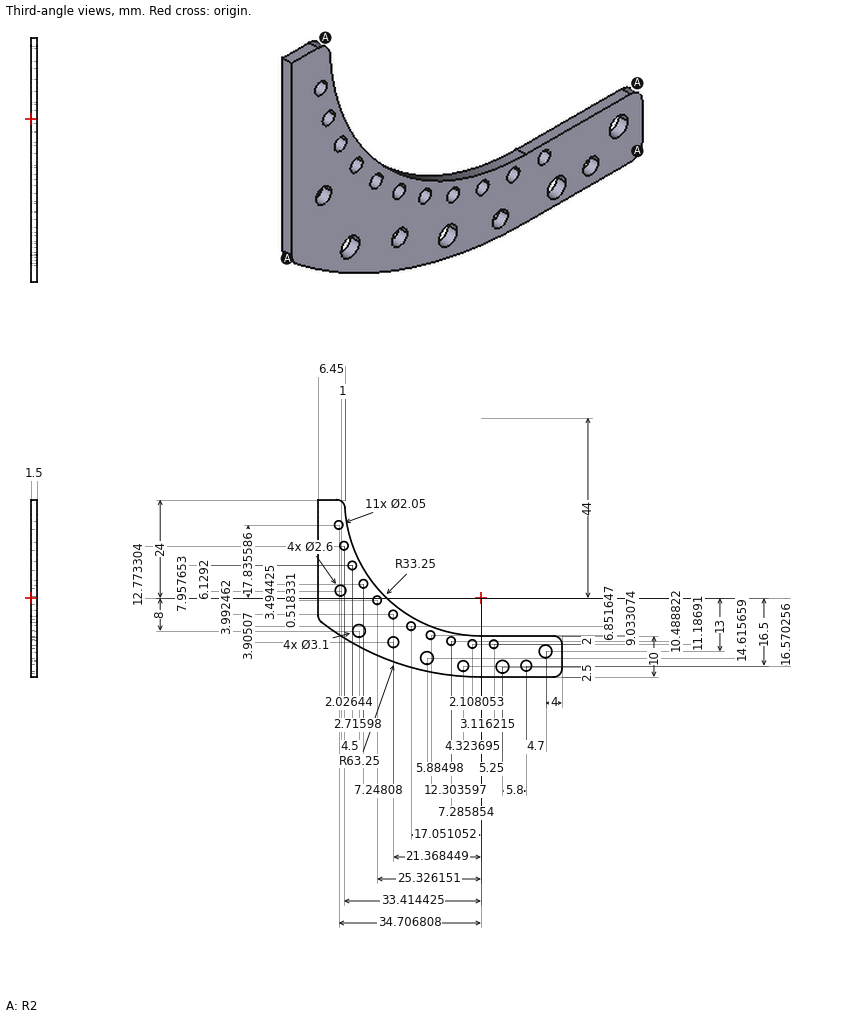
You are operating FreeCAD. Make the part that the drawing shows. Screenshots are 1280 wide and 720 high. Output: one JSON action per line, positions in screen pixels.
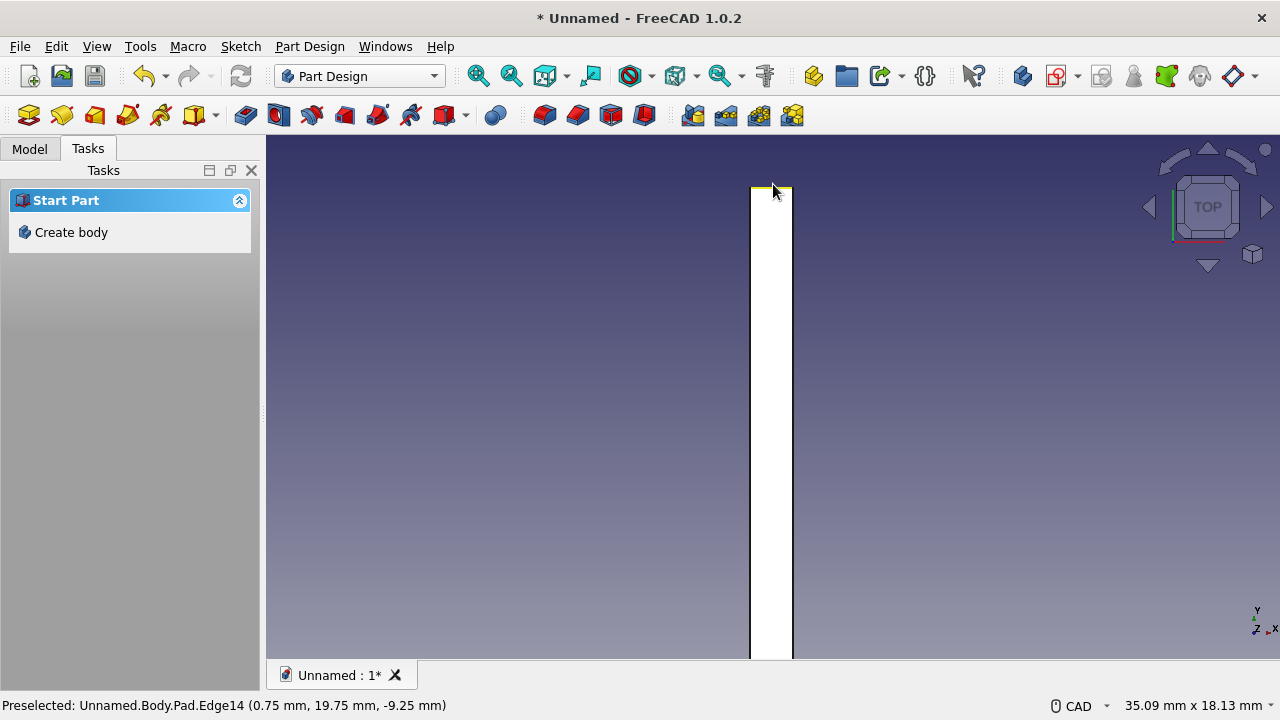
{"action": "left_click", "coordinate": [771, 187]}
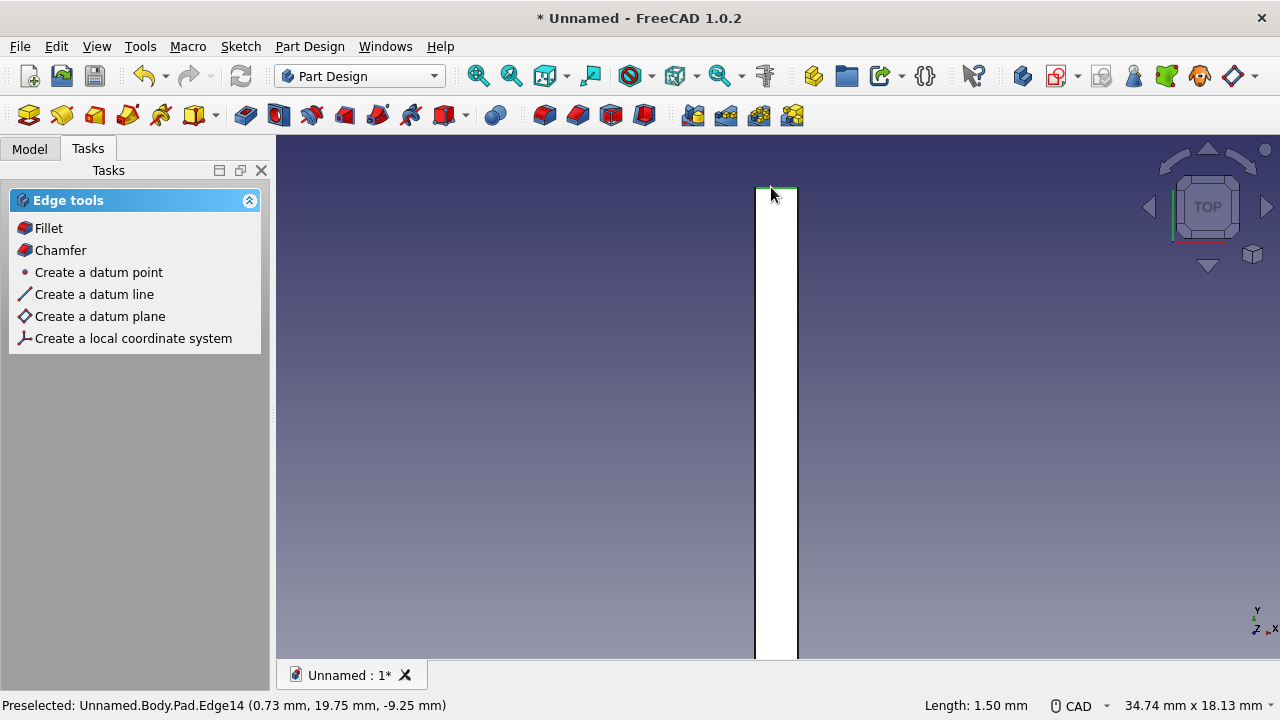
{"action": "left_click", "coordinate": [479, 76]}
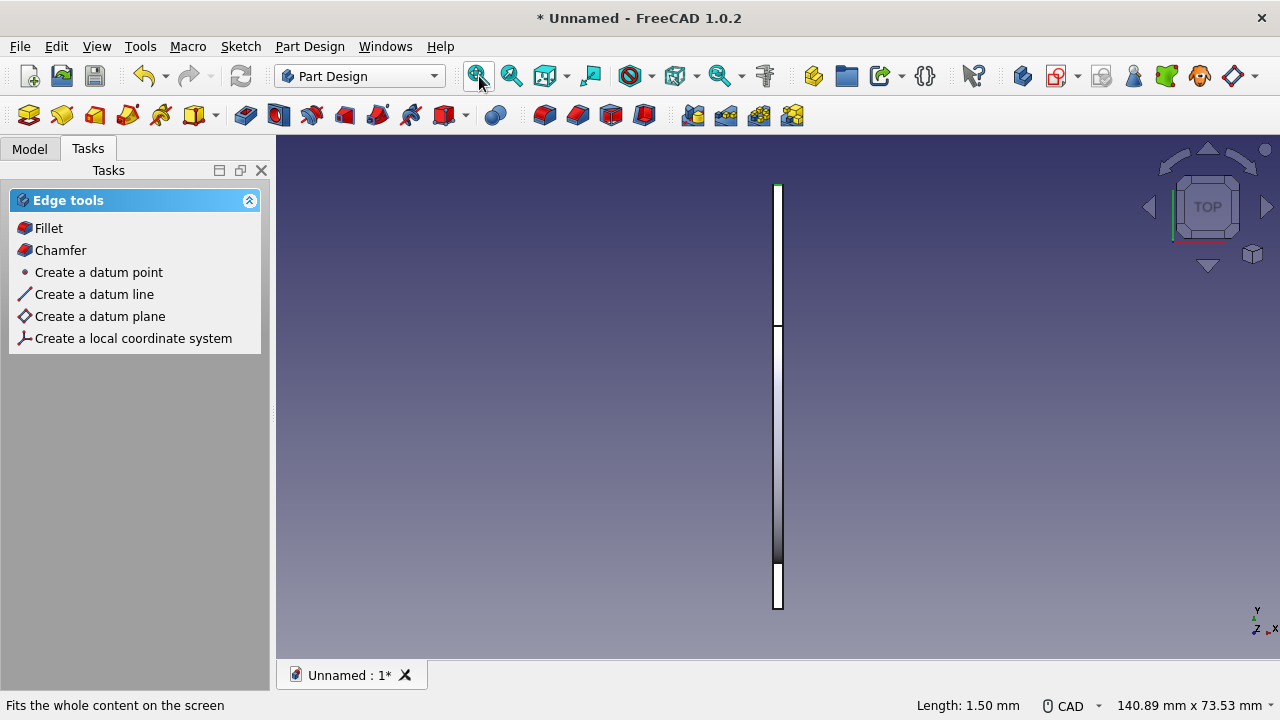
{"action": "key", "text": "1"}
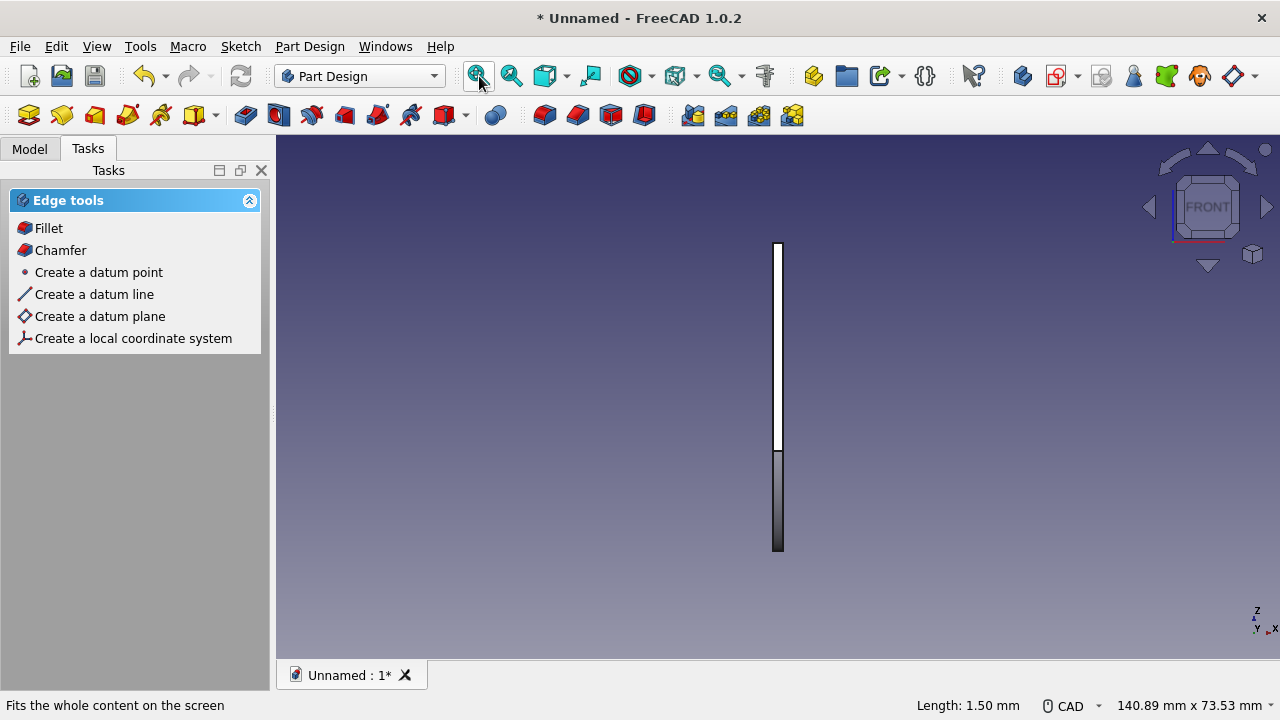
{"action": "scroll", "coordinate": [778, 550], "scroll_direction": "up", "scroll_amount": 7}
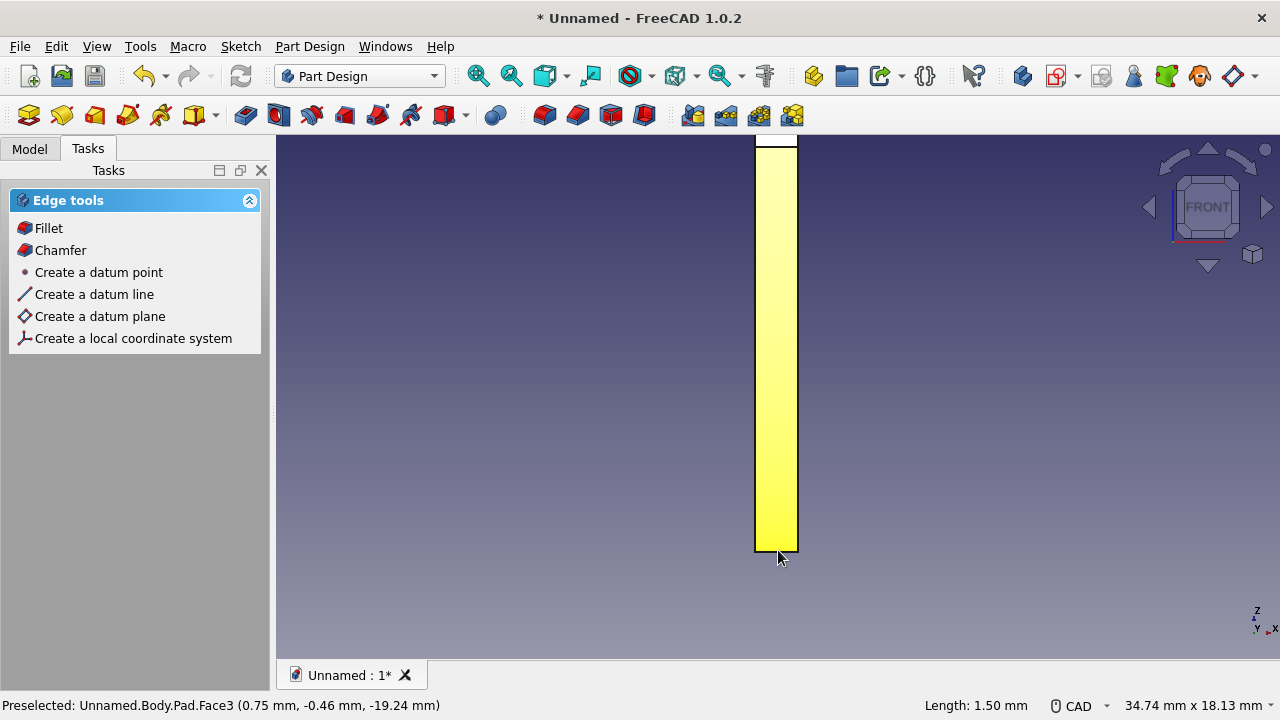
{"action": "left_click", "coordinate": [479, 76]}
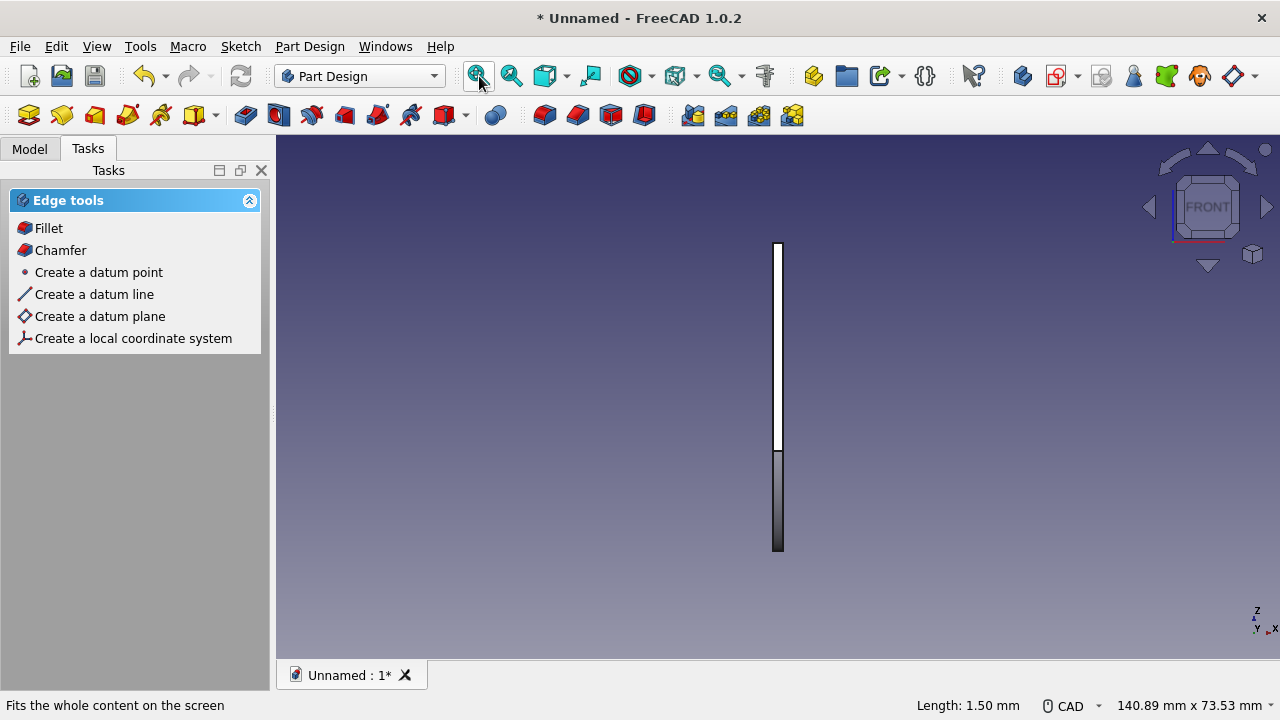
{"action": "key", "text": "3"}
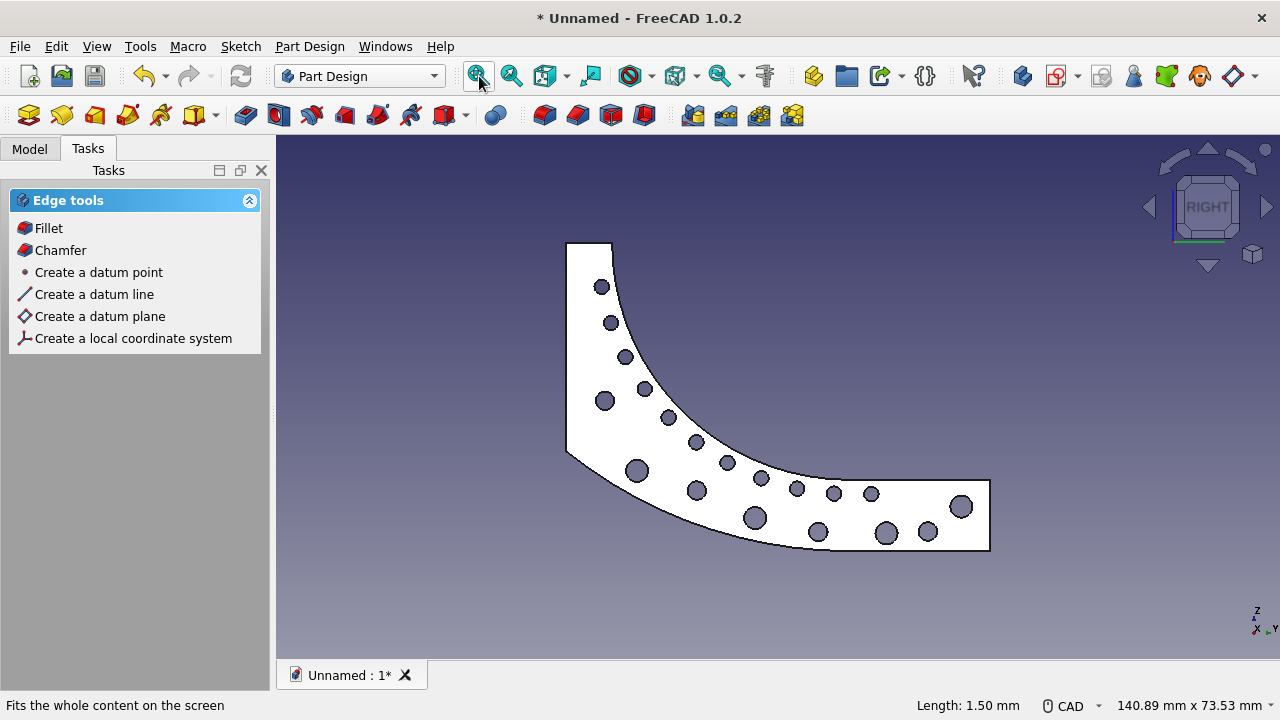
{"action": "scroll", "coordinate": [990, 550], "scroll_direction": "up", "scroll_amount": 7}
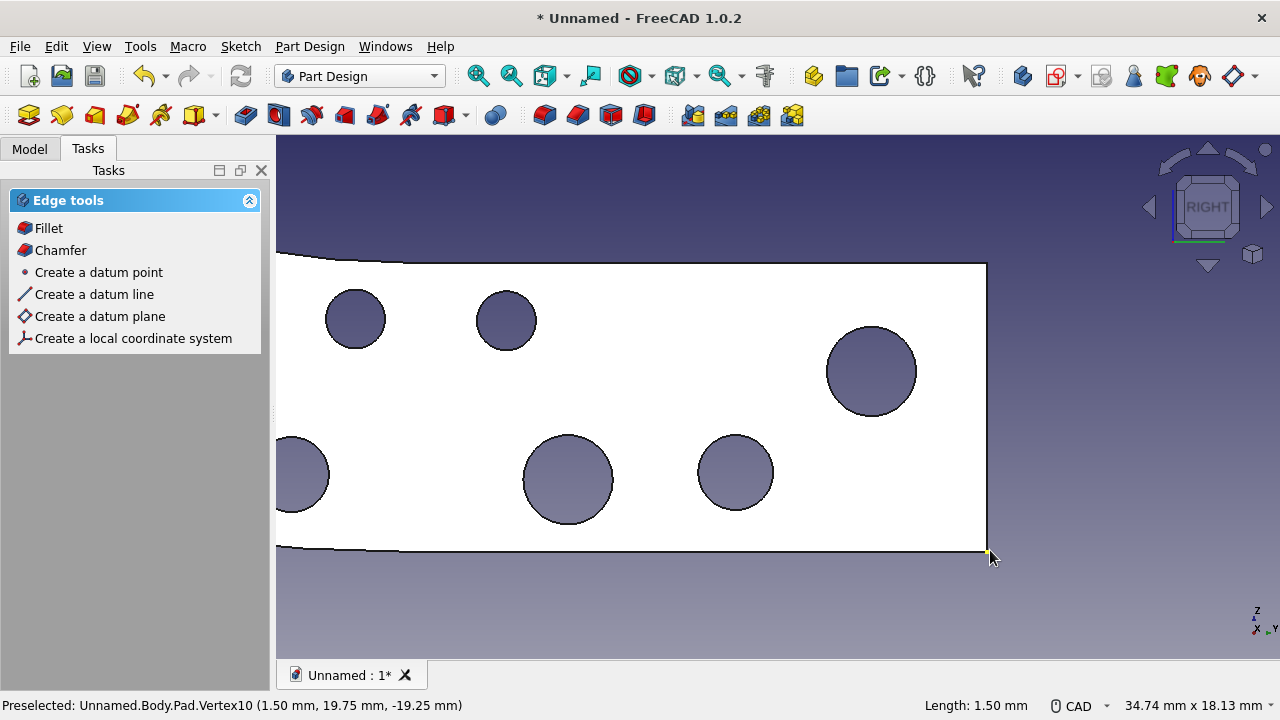
{"action": "left_click", "coordinate": [479, 76]}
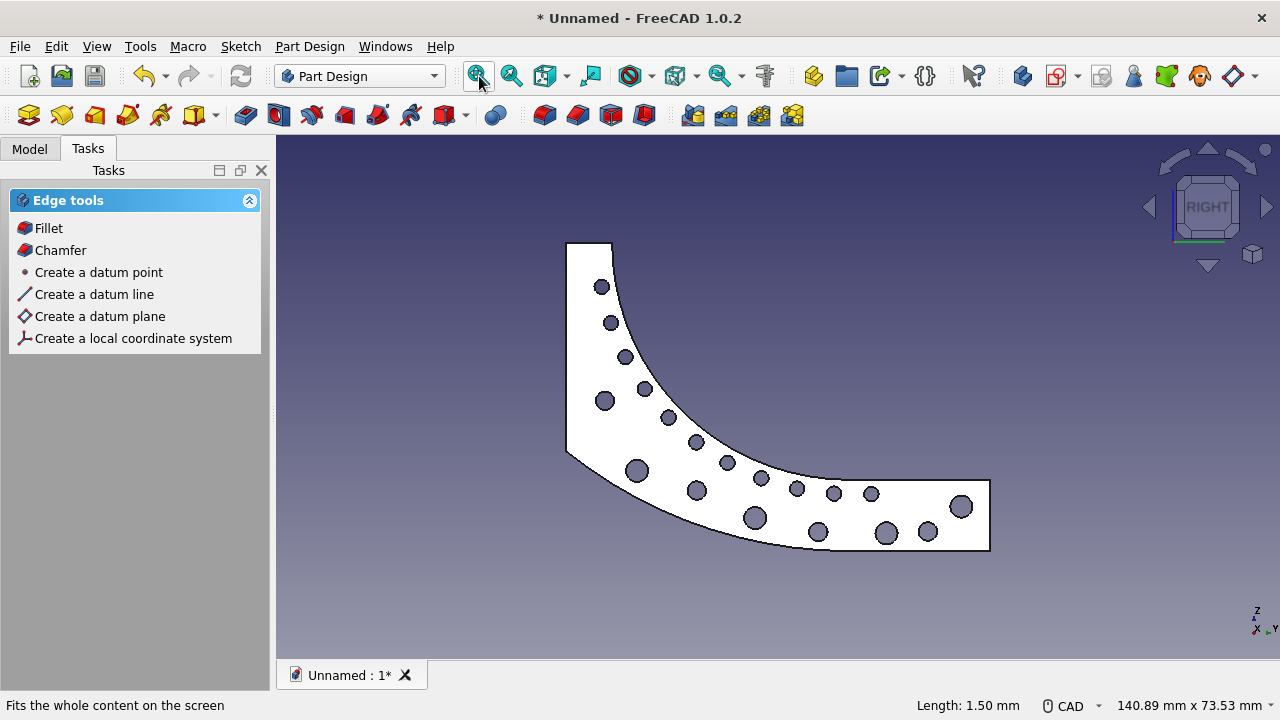
{"action": "key", "text": "5"}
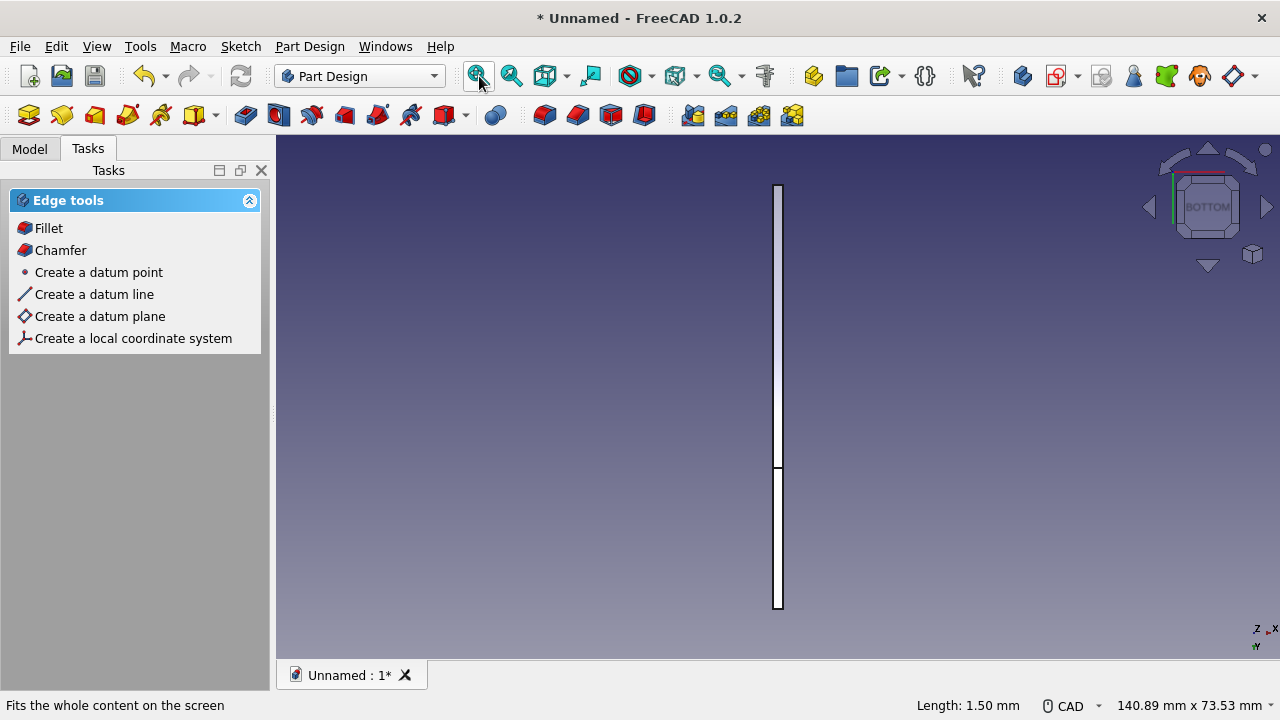
{"action": "scroll", "coordinate": [778, 608], "scroll_direction": "up", "scroll_amount": 7}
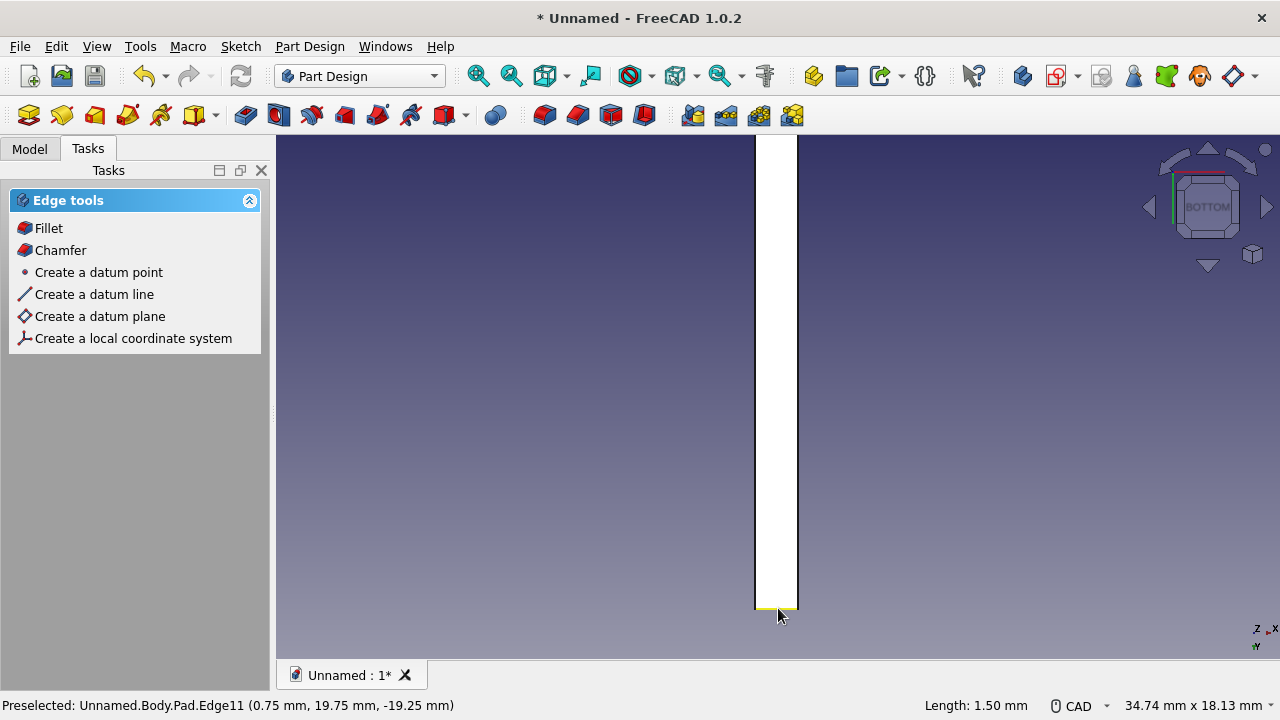
{"action": "left_click", "coordinate": [776, 608], "text": "ctrl"}